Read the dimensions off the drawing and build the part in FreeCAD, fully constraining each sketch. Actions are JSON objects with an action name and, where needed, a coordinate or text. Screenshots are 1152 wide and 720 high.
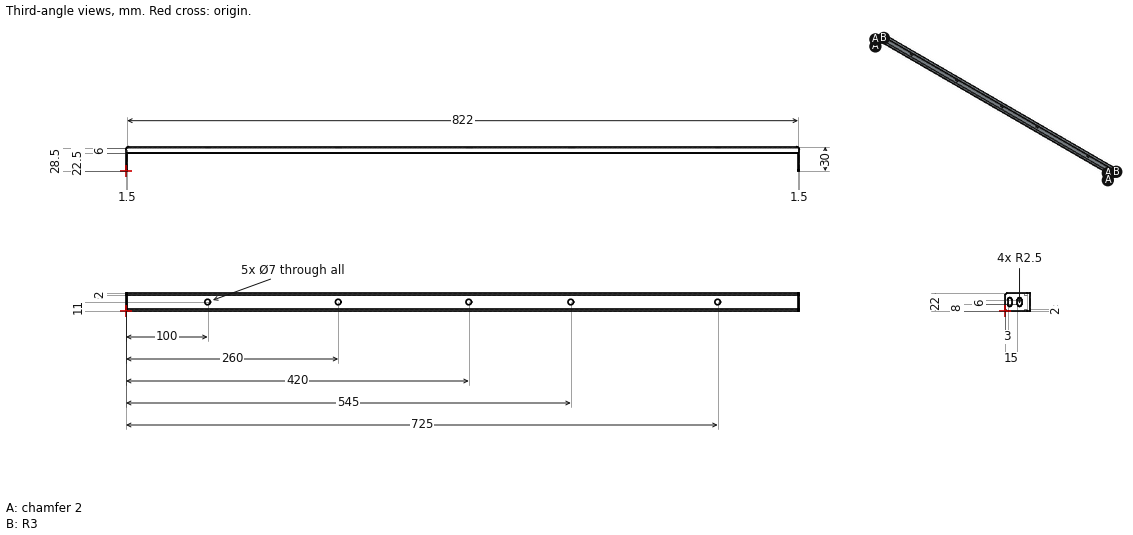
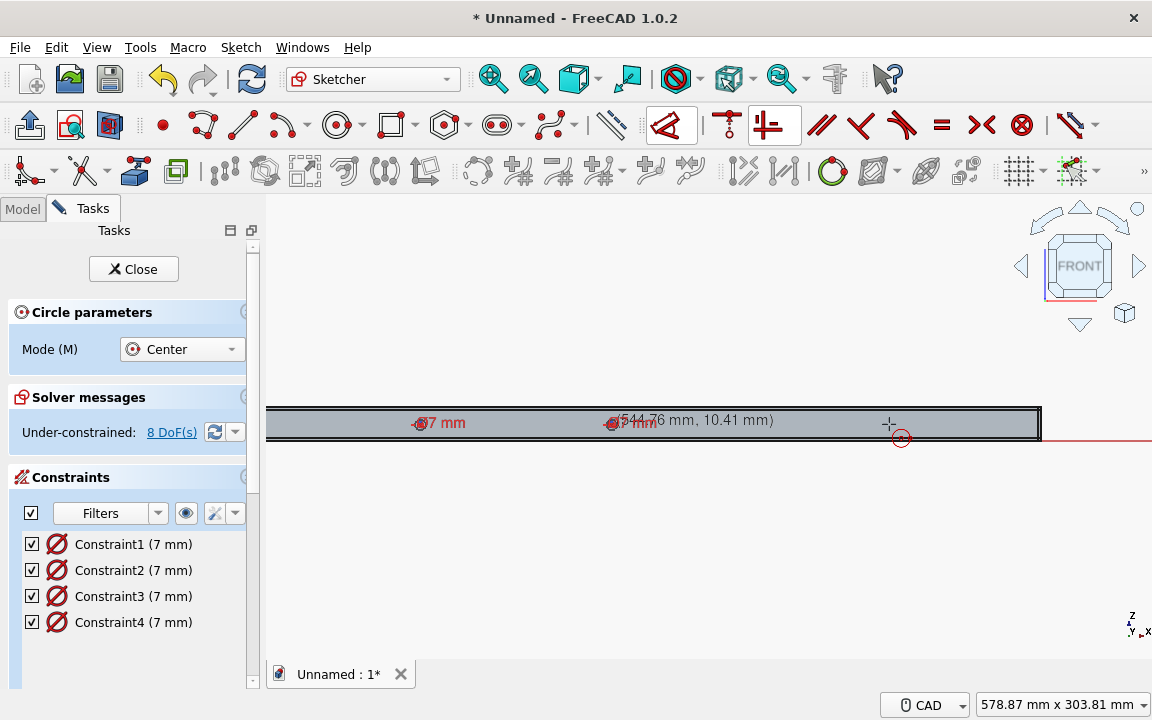
{"action": "left_click", "coordinate": [888, 424]}
{"action": "mouse_move", "coordinate": [892, 420]}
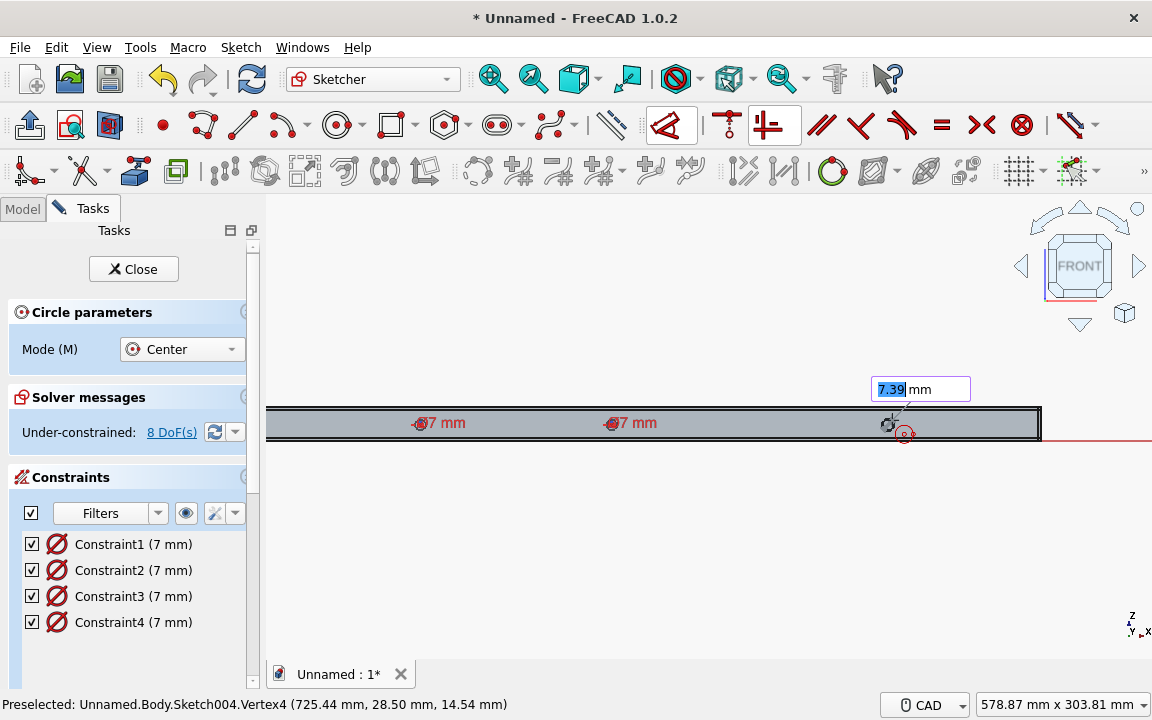
{"action": "type", "text": "7"}
{"action": "key", "text": "Return"}
{"action": "key", "text": "Escape"}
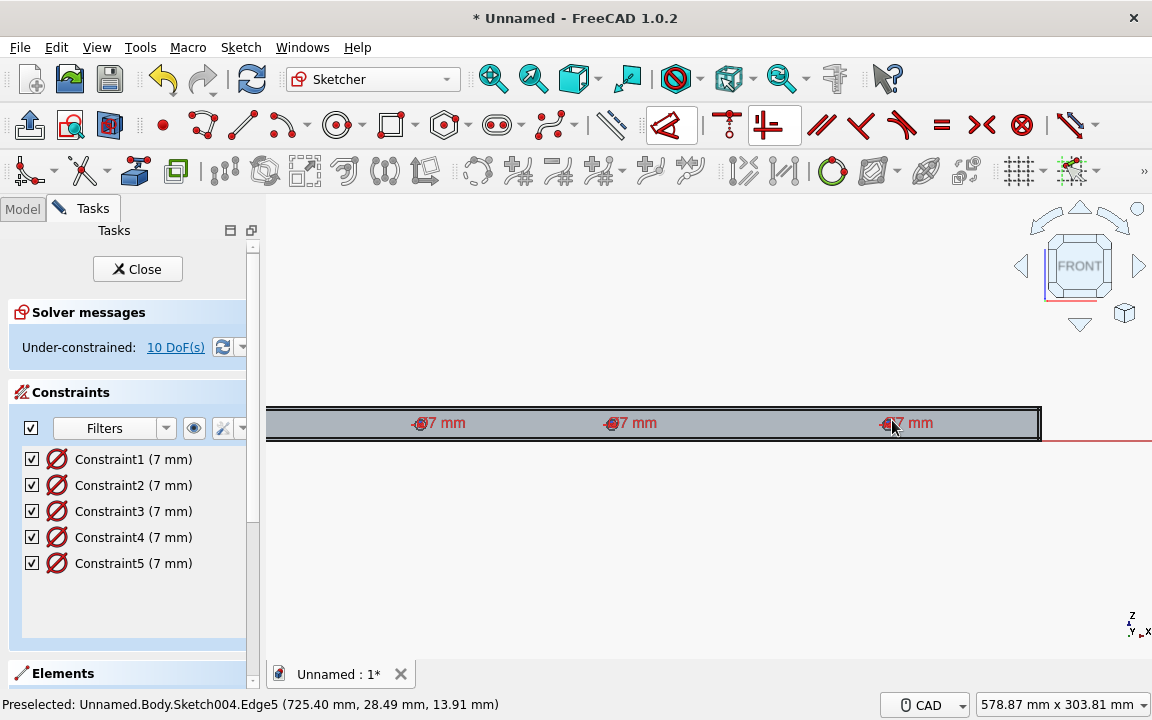
{"action": "scroll", "coordinate": [889, 424], "scroll_direction": "down", "scroll_amount": 4}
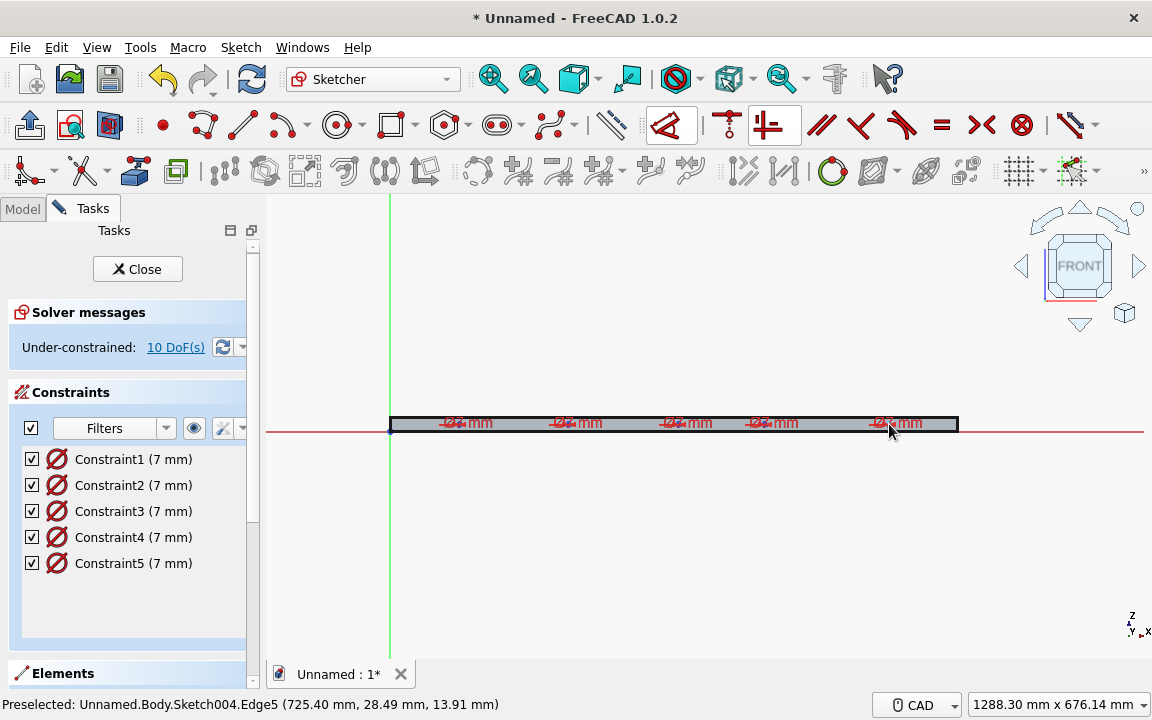
{"action": "scroll", "coordinate": [459, 425], "scroll_direction": "up", "scroll_amount": 9}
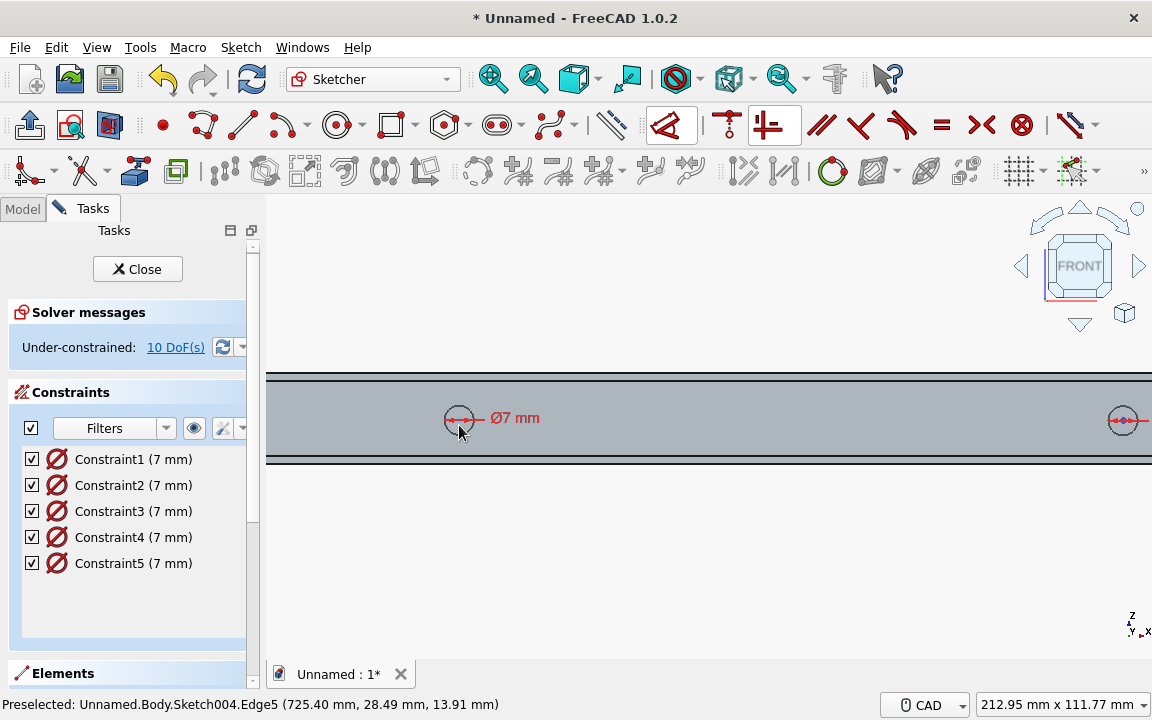
{"action": "left_click", "coordinate": [459, 420]}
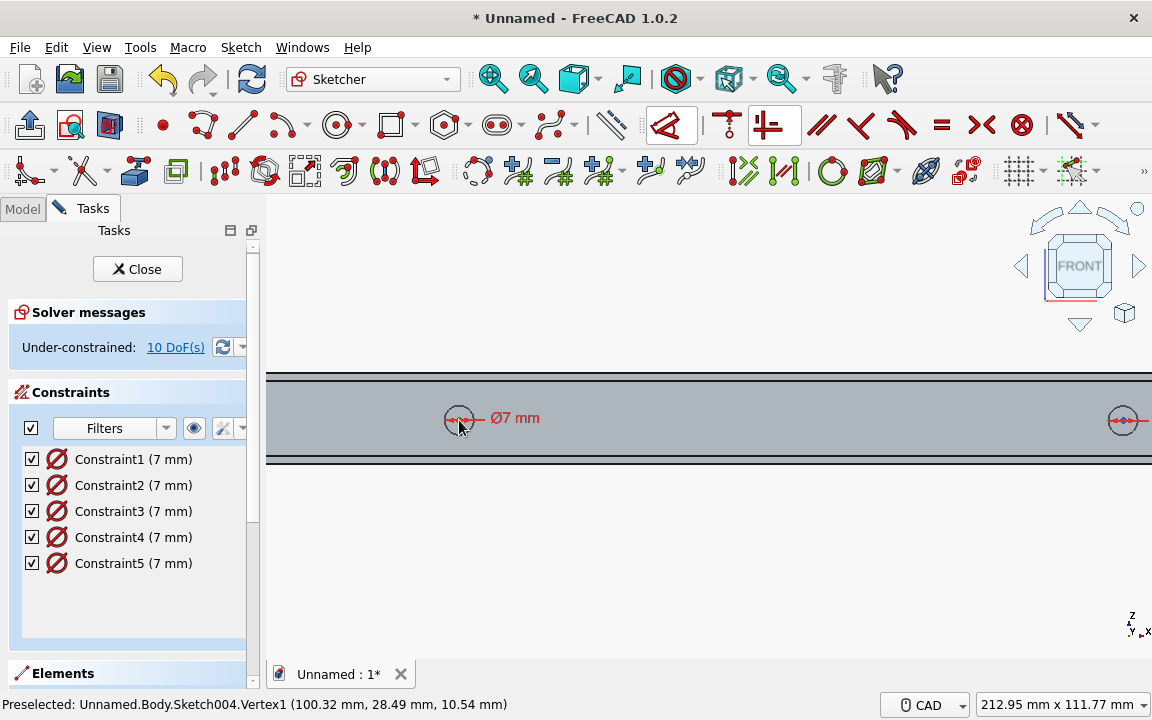
{"action": "left_click", "coordinate": [692, 126]}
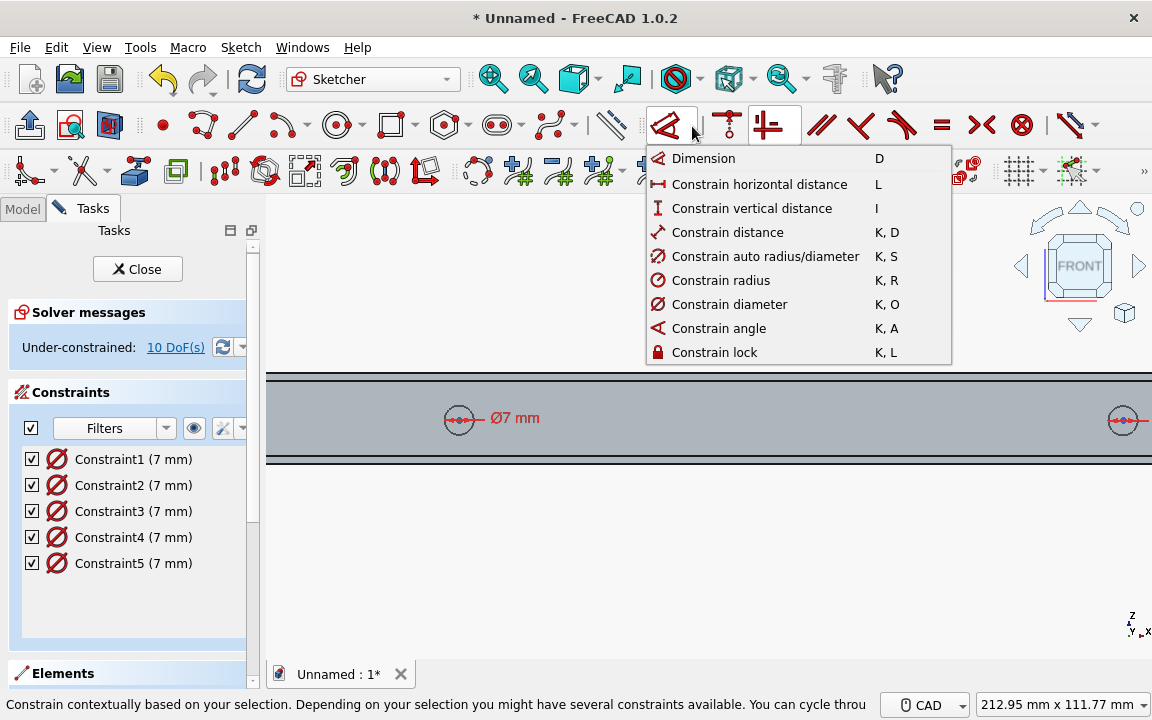
{"action": "left_click", "coordinate": [799, 208]}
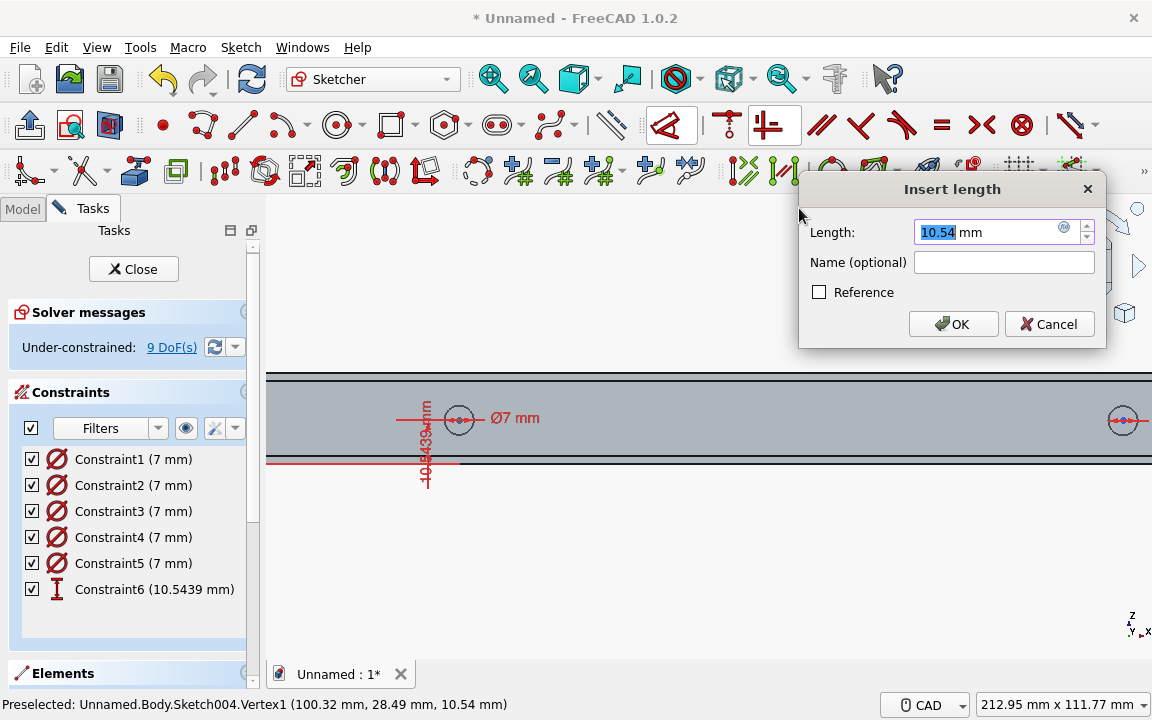
{"action": "type", "text": "11"}
{"action": "key", "text": "Return"}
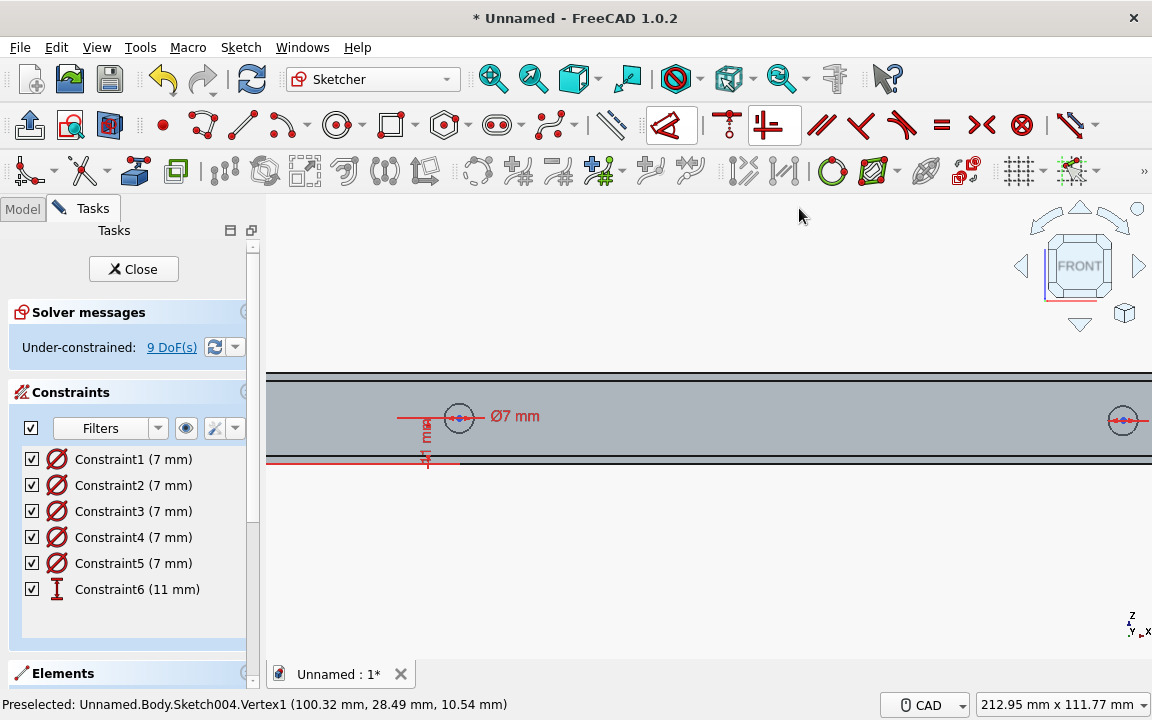
{"action": "scroll", "coordinate": [459, 425], "scroll_direction": "down", "scroll_amount": 9}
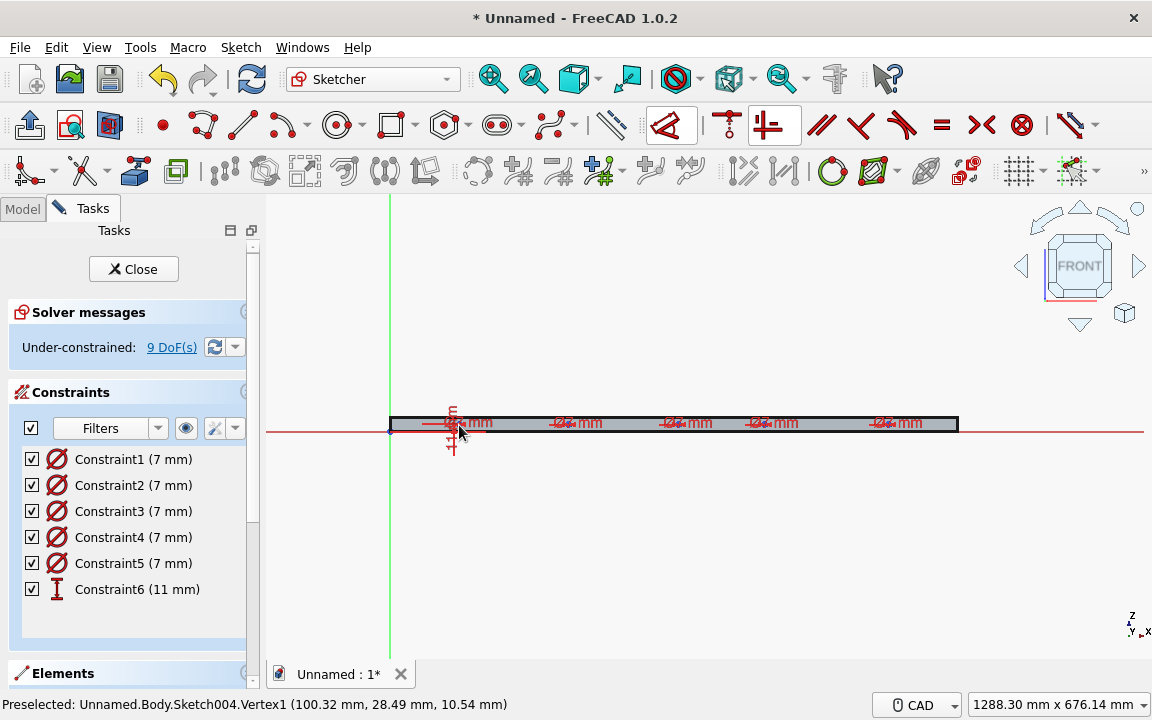
{"action": "scroll", "coordinate": [569, 425], "scroll_direction": "up", "scroll_amount": 9}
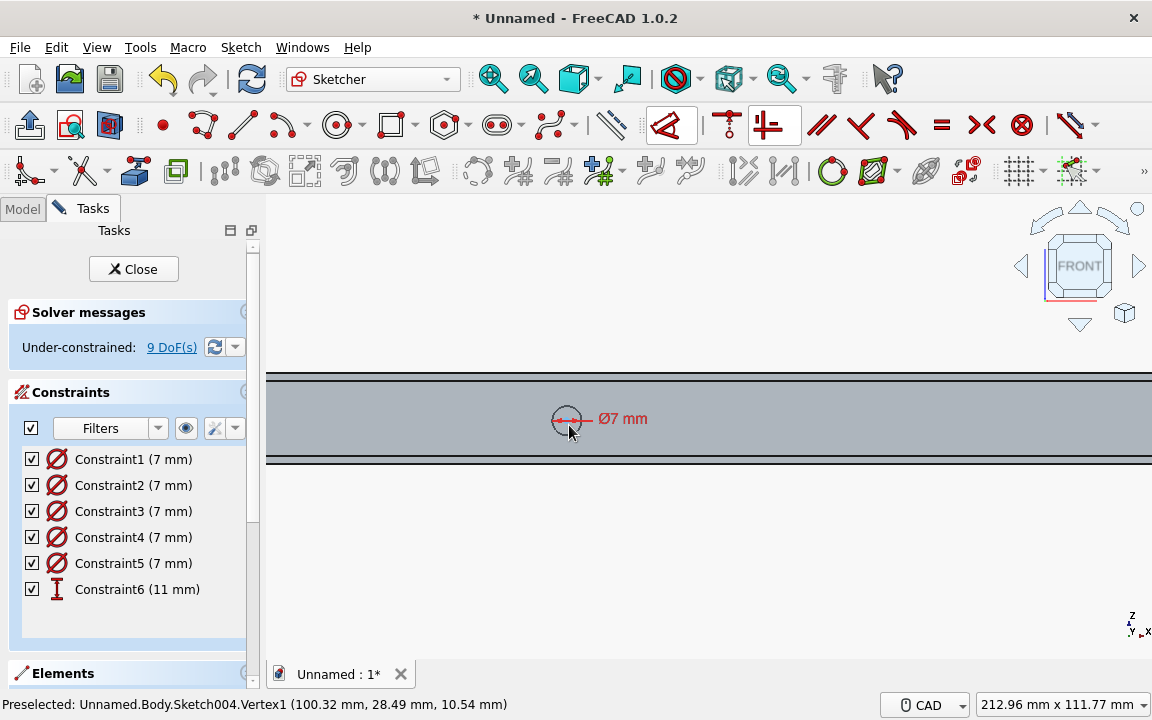
{"action": "left_click", "coordinate": [567, 421]}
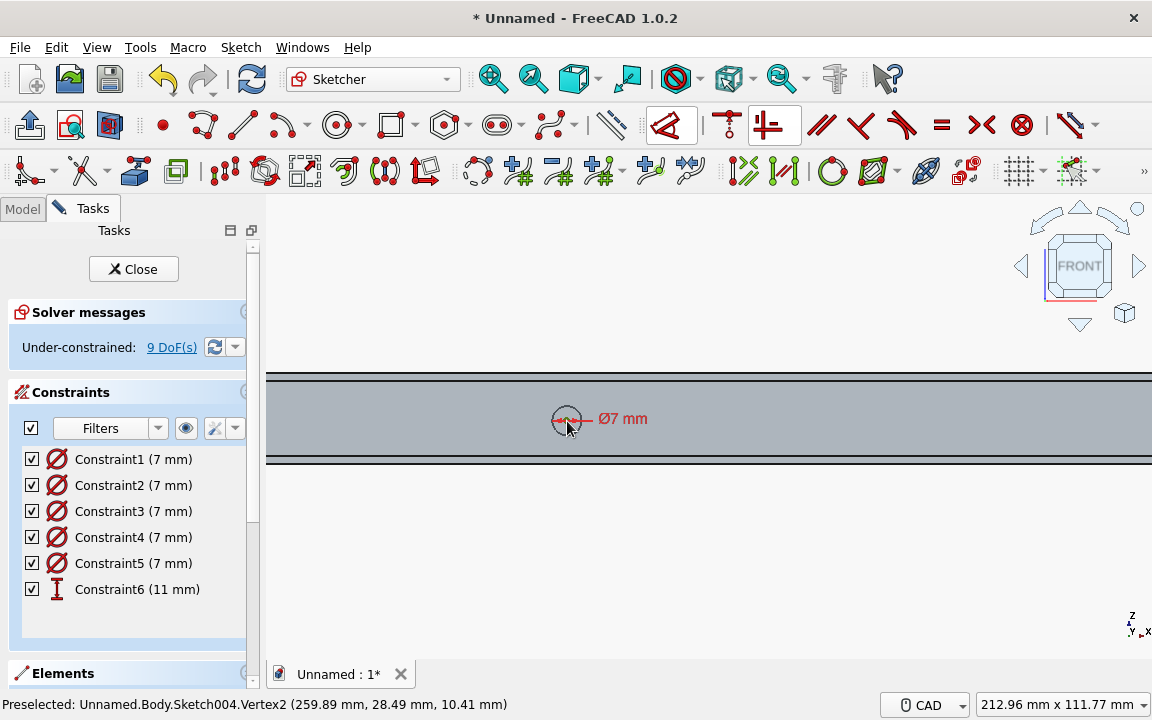
{"action": "left_click", "coordinate": [692, 126]}